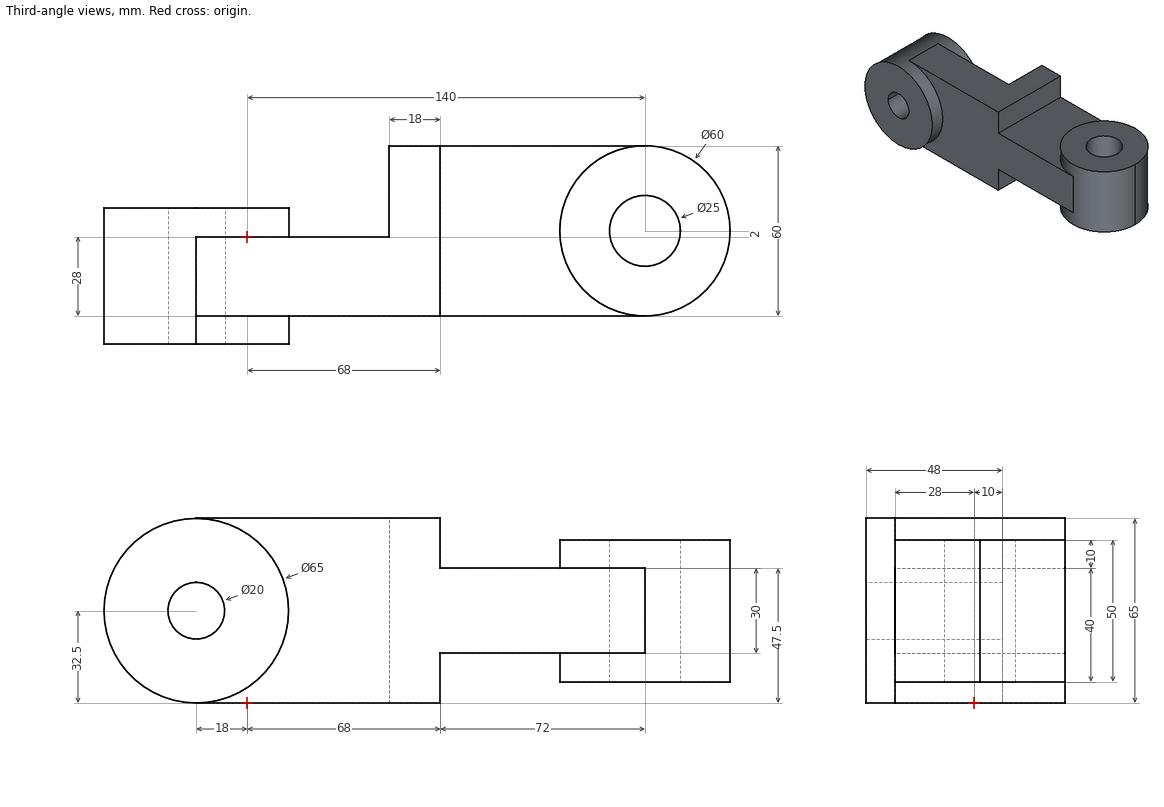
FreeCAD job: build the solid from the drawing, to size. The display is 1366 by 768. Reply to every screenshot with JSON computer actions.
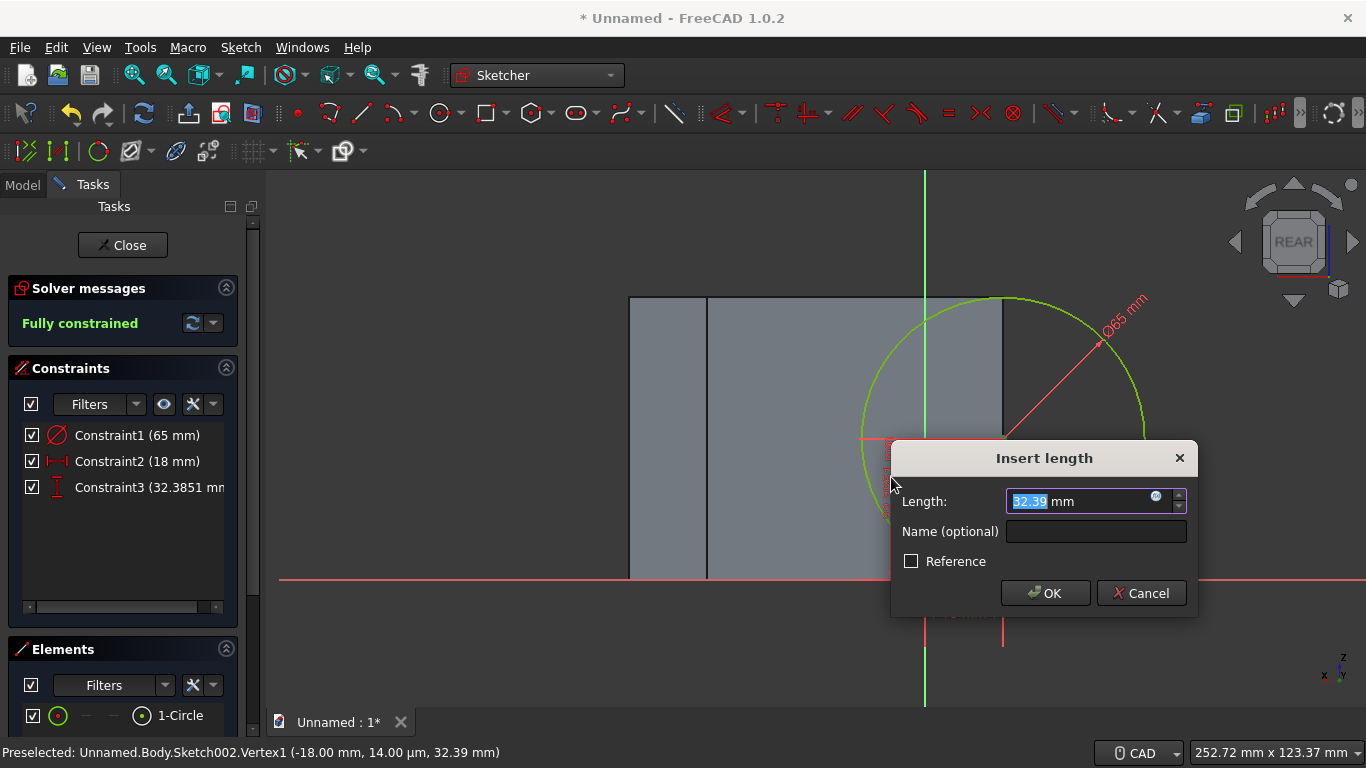
{"action": "type", "text": "32.5"}
{"action": "key", "text": "Return"}
{"action": "key", "text": "Escape"}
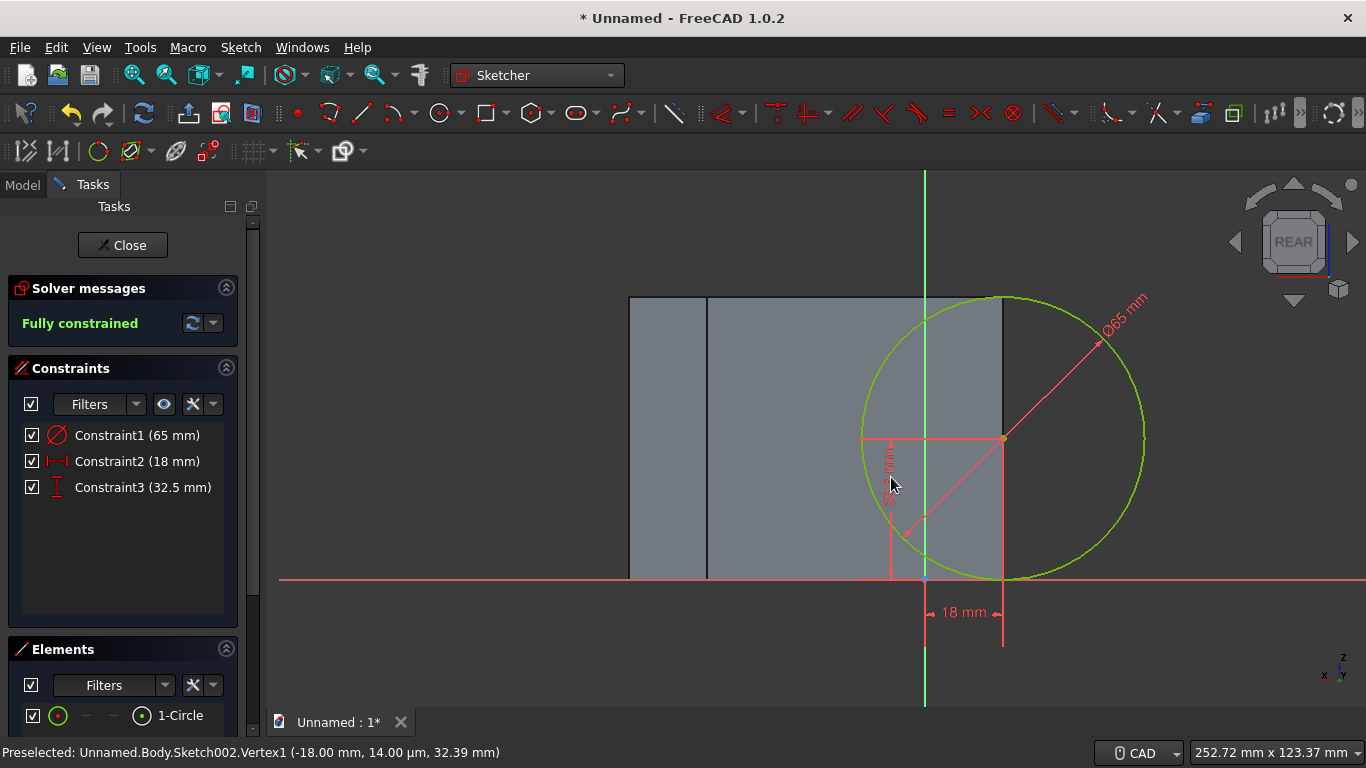
{"action": "left_click", "coordinate": [123, 245]}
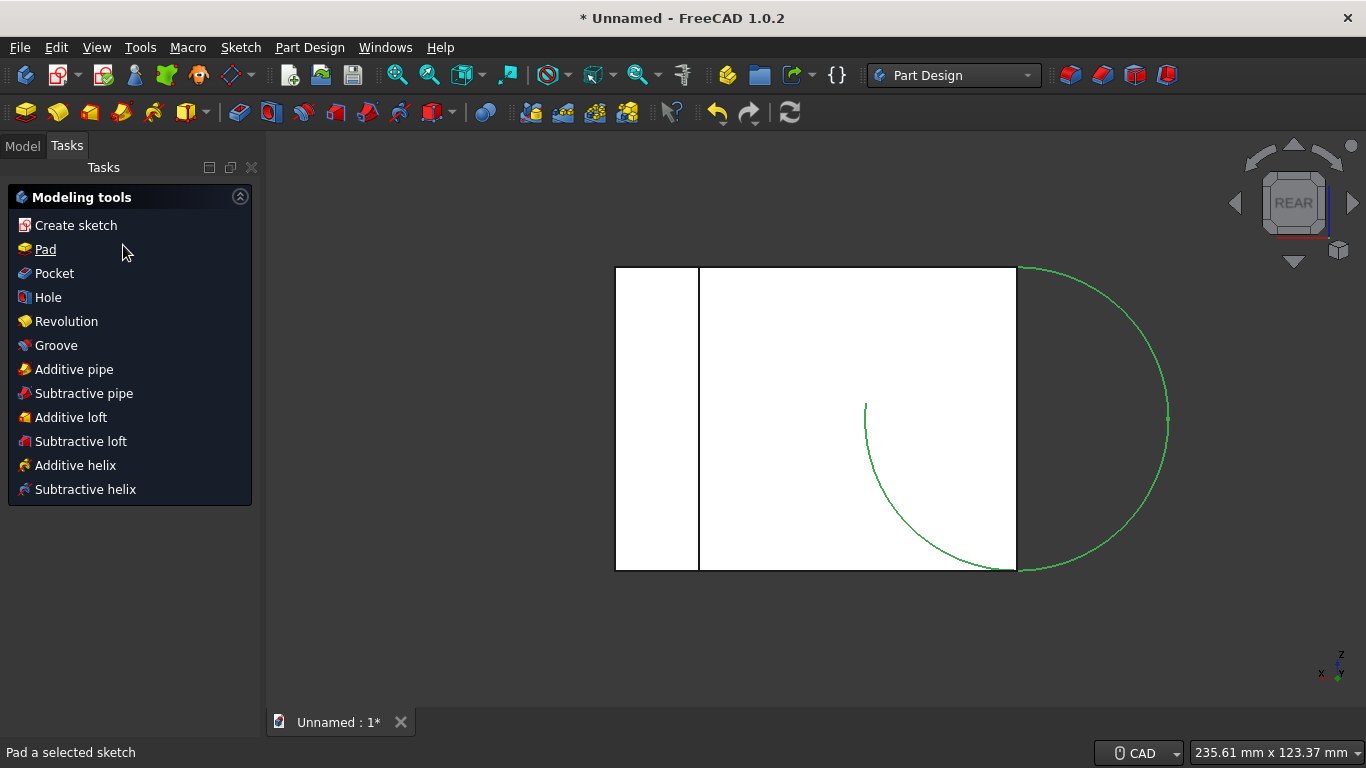
{"action": "left_click", "coordinate": [26, 112]}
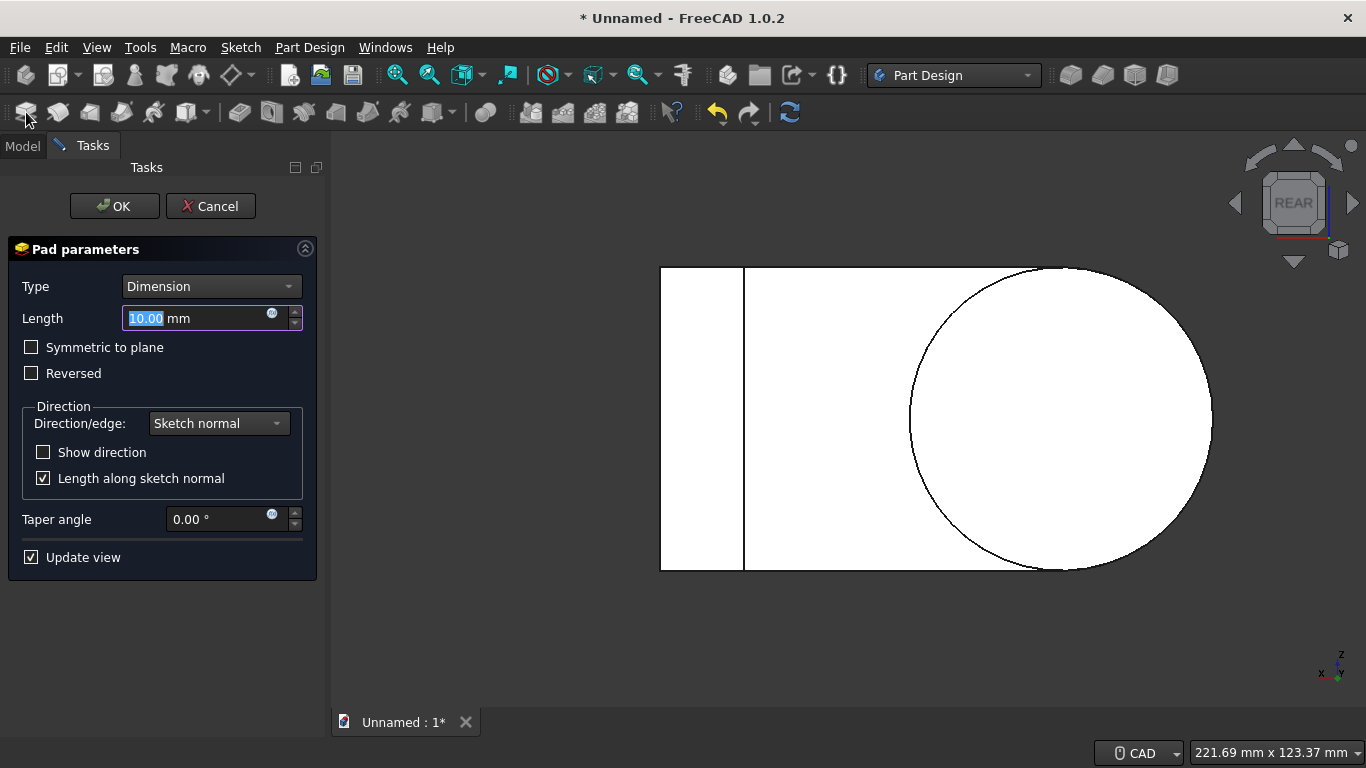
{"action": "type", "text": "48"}
{"action": "key", "text": "Tab"}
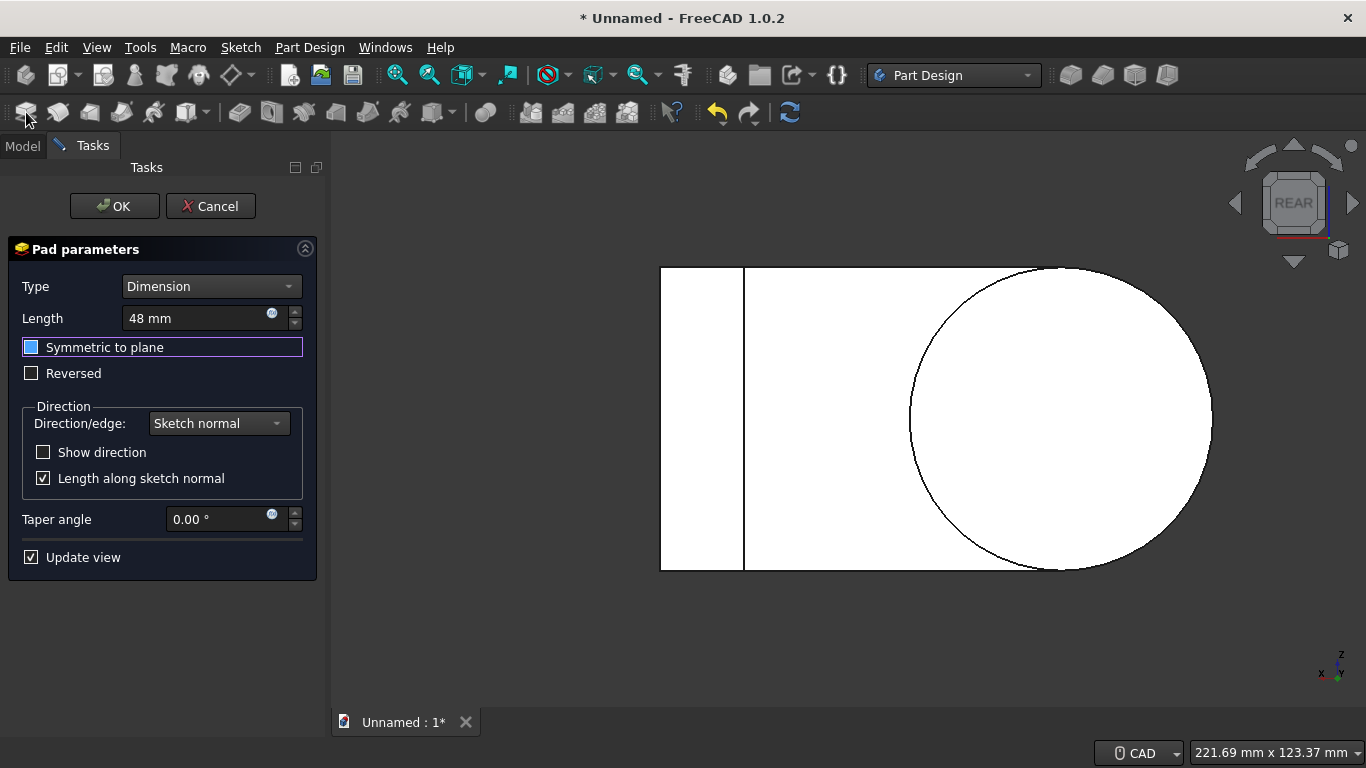
{"action": "left_click", "coordinate": [30, 373]}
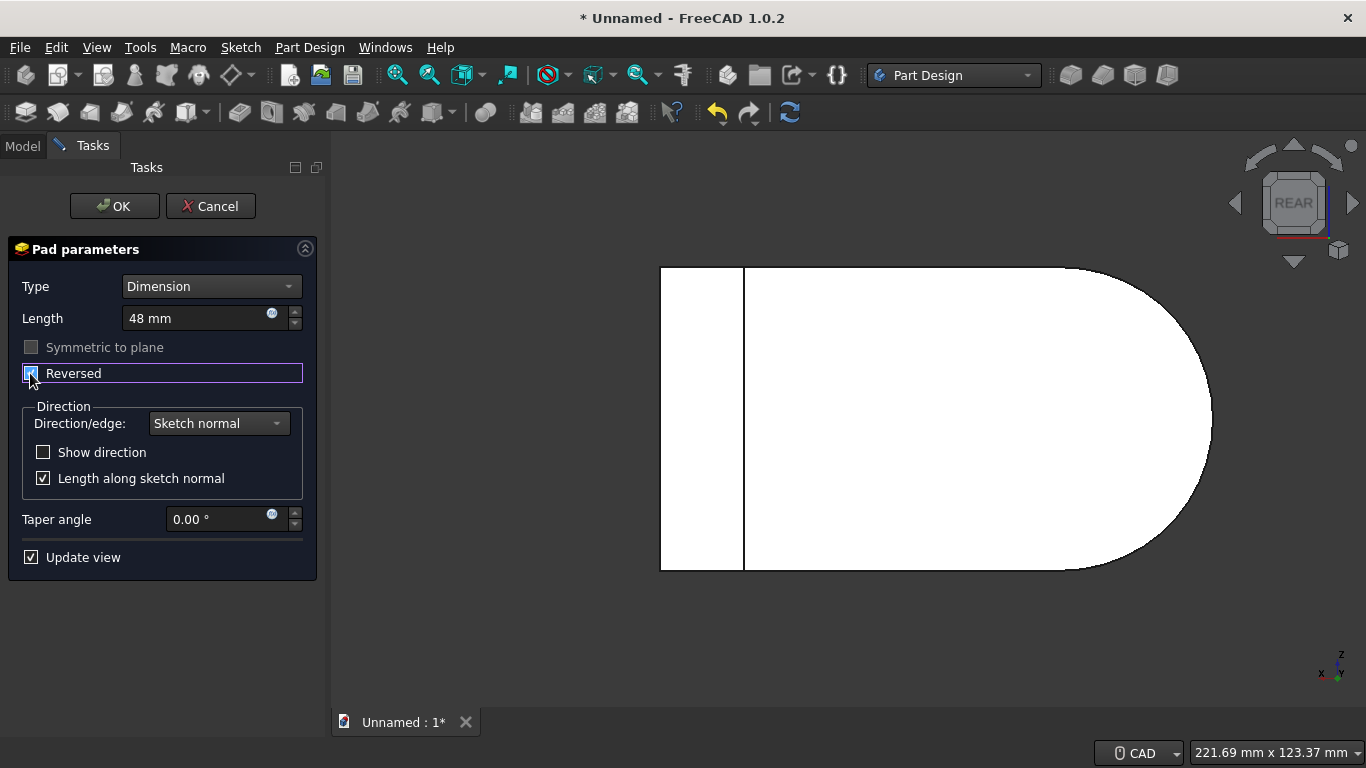
{"action": "left_click", "coordinate": [115, 206]}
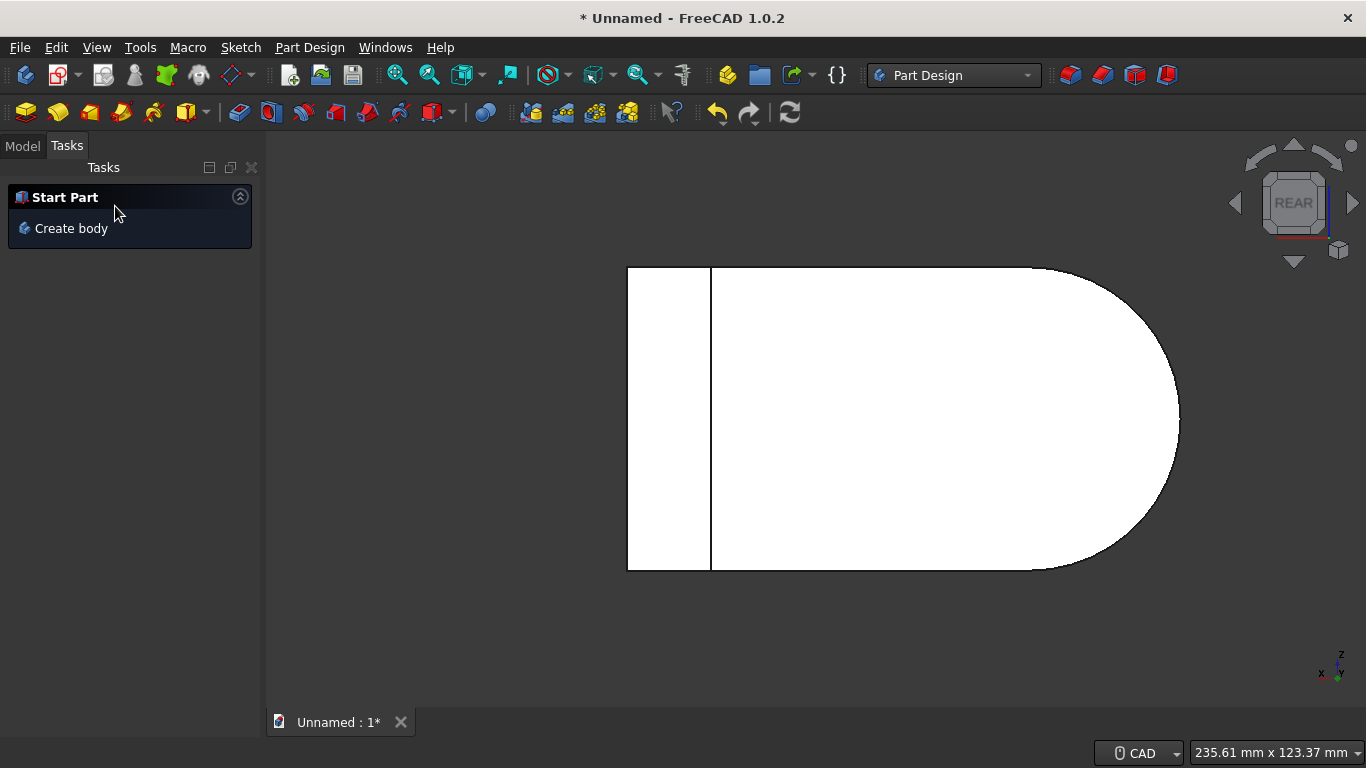
{"action": "left_click", "coordinate": [23, 145]}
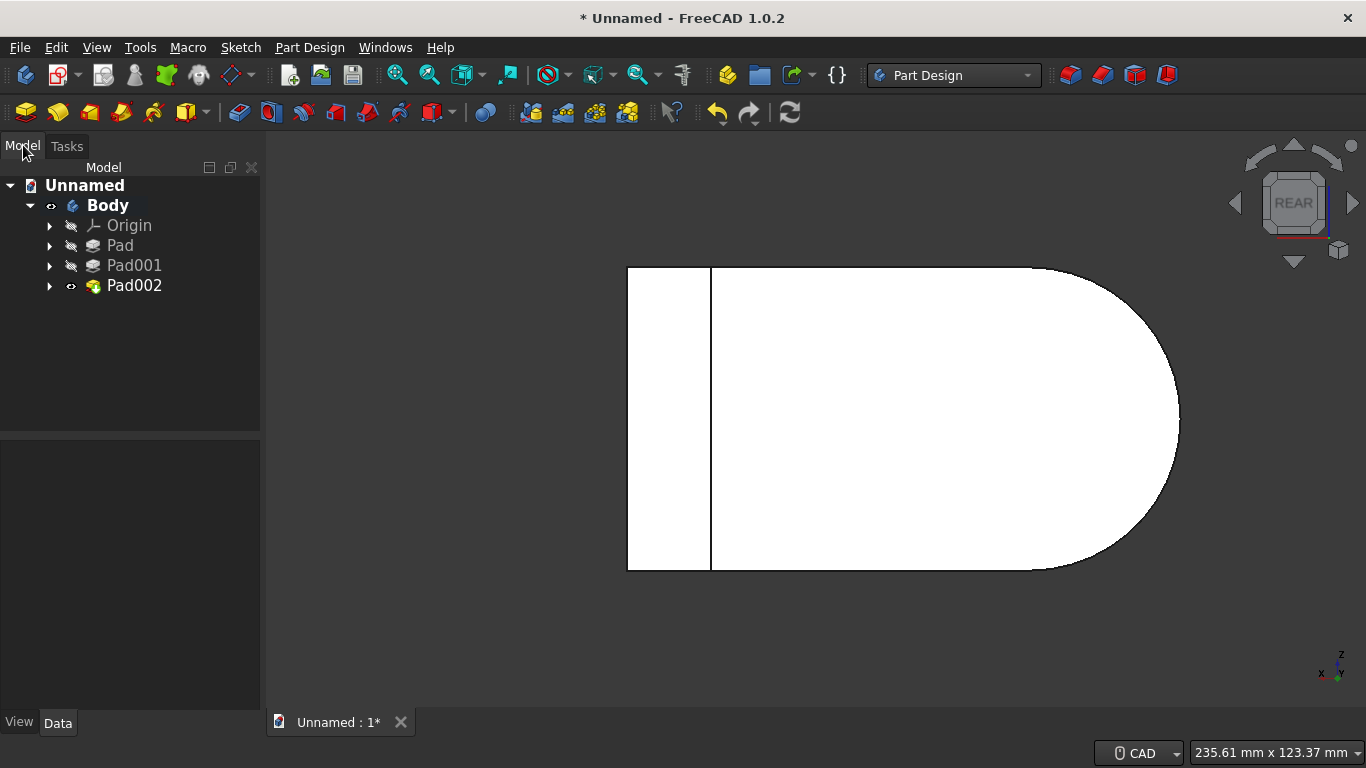
{"action": "left_click", "coordinate": [50, 226]}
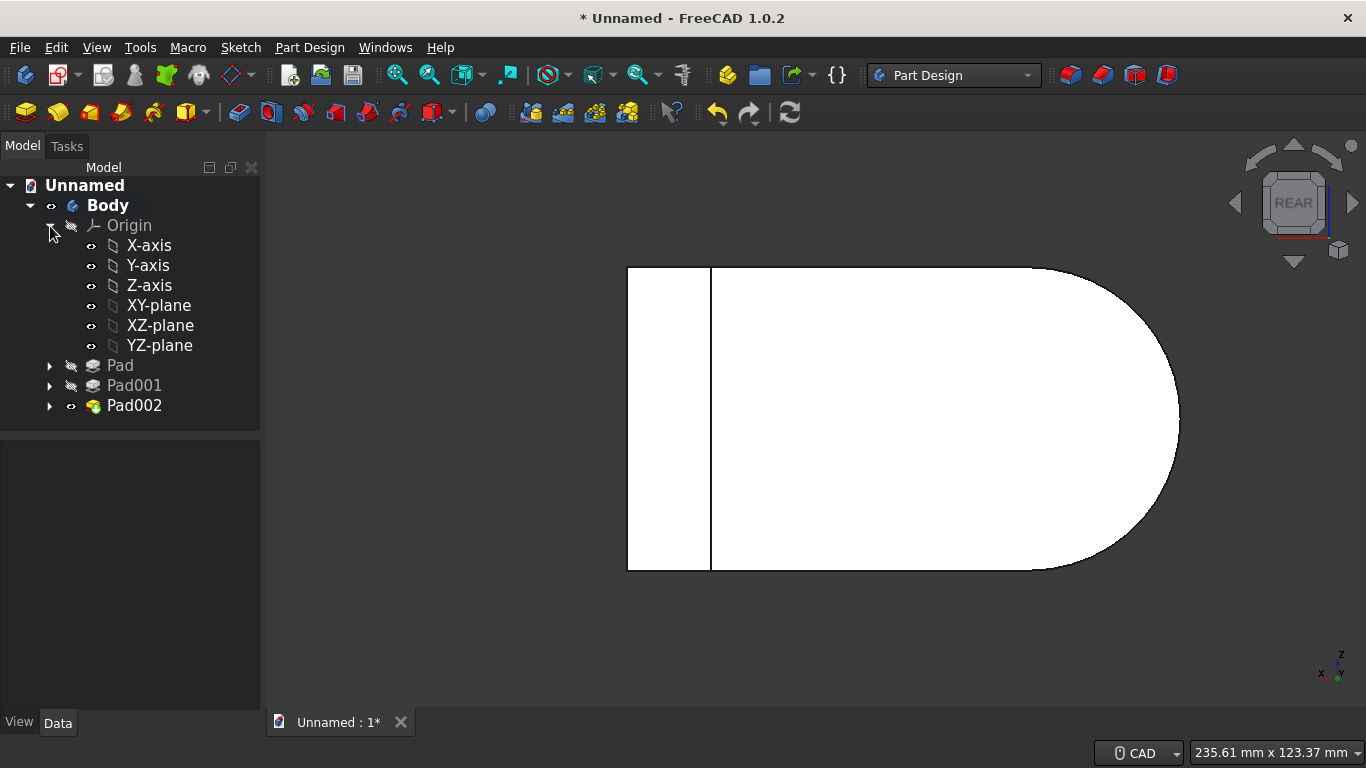
{"action": "left_click", "coordinate": [136, 326]}